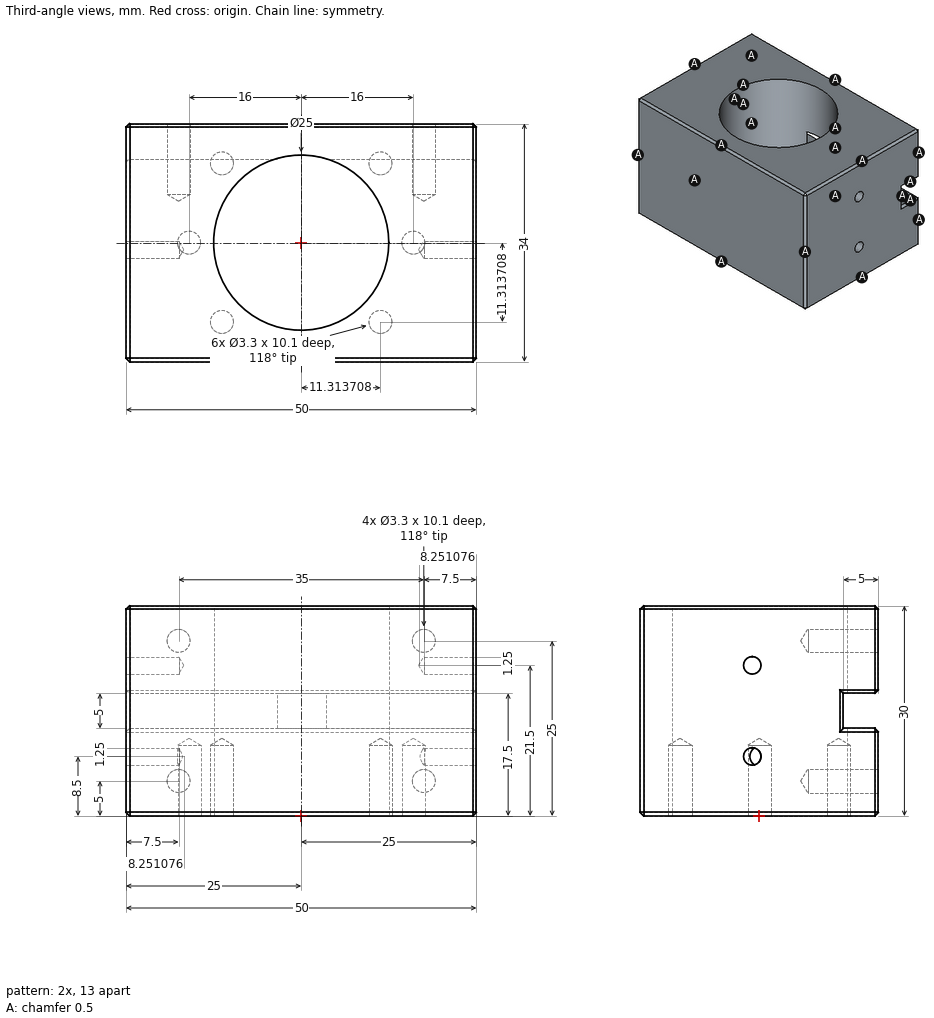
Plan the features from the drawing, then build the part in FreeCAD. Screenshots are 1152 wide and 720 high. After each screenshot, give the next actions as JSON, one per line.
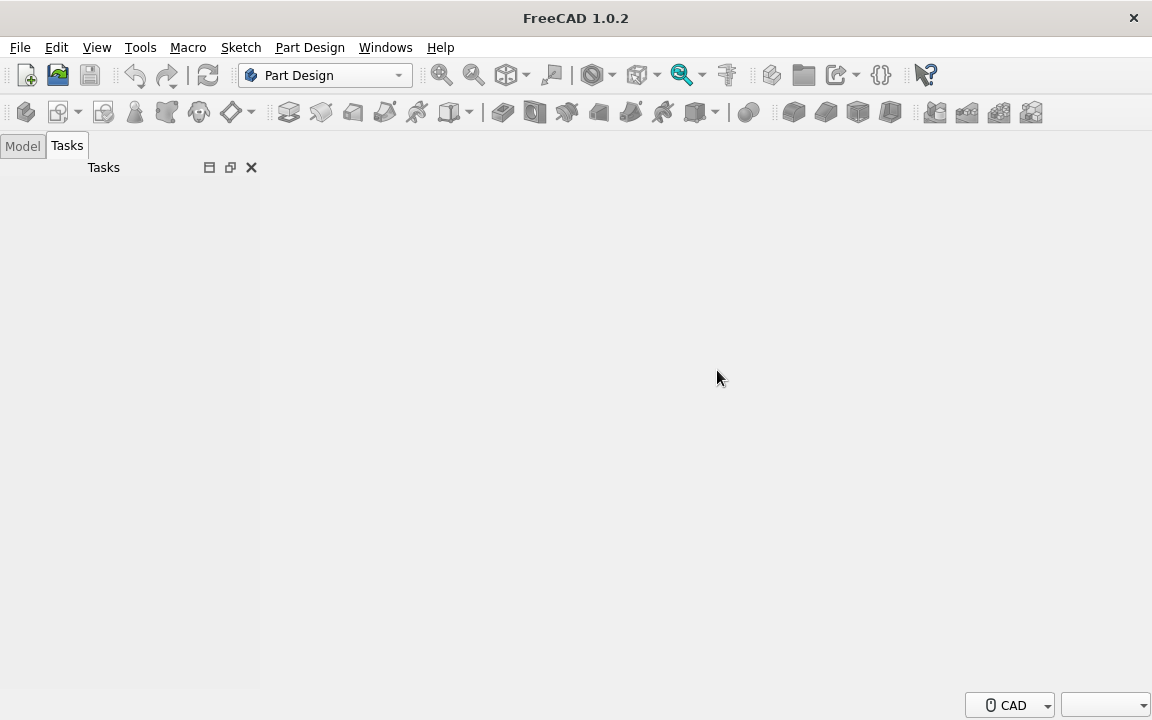
{"action": "key", "text": "ctrl+n"}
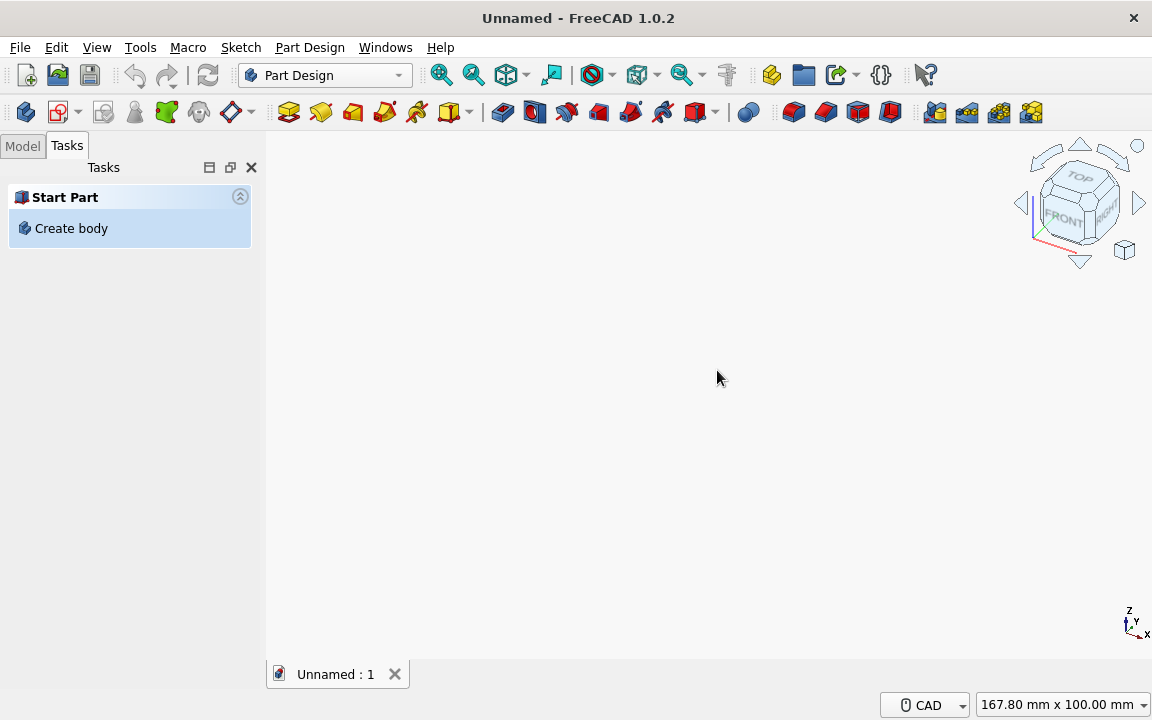
{"action": "left_click", "coordinate": [58, 112]}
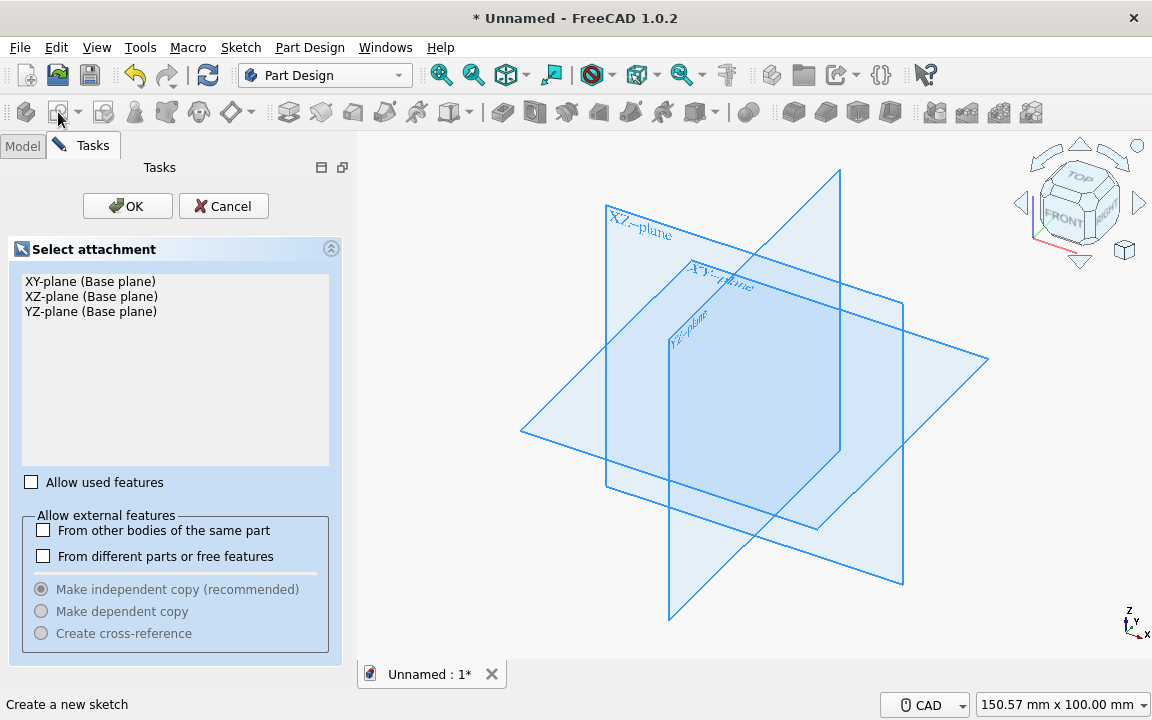
{"action": "left_click", "coordinate": [82, 282]}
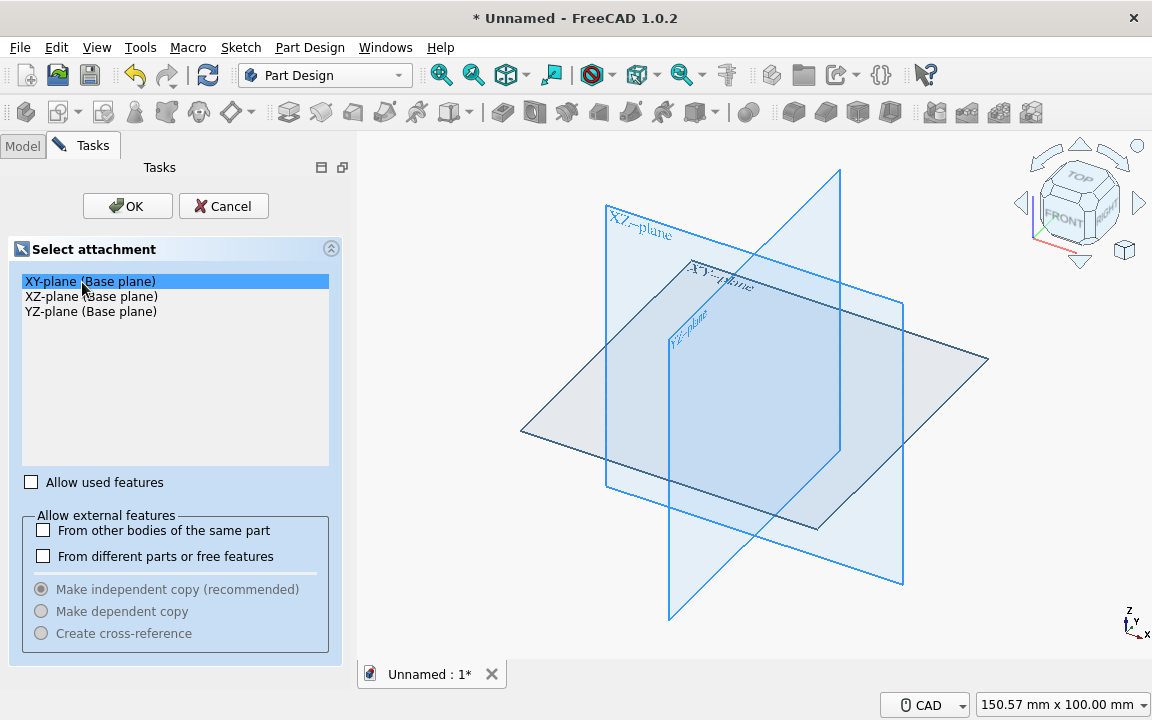
{"action": "left_click", "coordinate": [128, 206]}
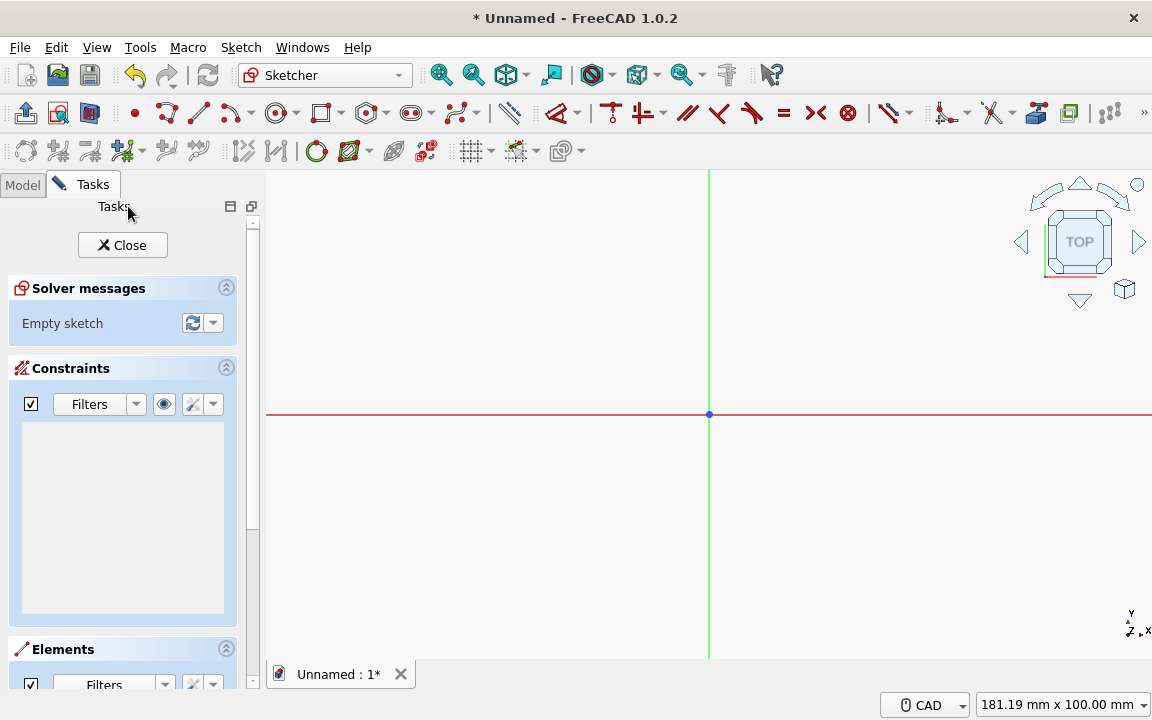
{"action": "scroll", "coordinate": [792, 415], "scroll_direction": "up", "scroll_amount": 3}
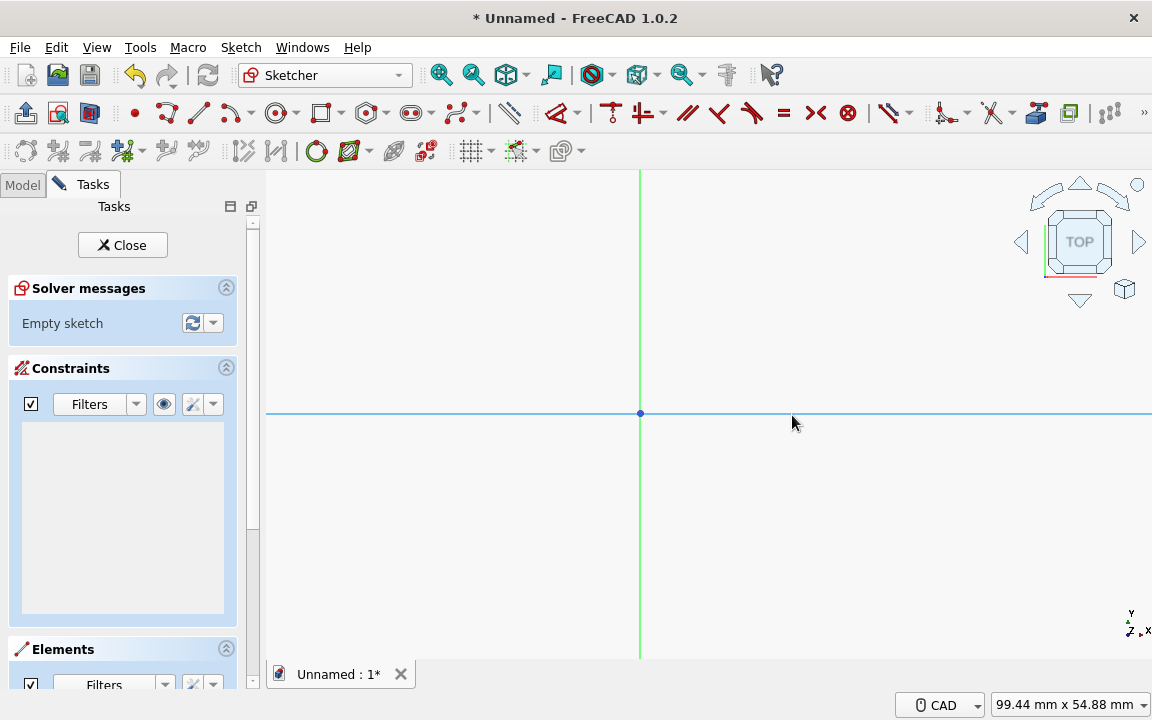
{"action": "left_click", "coordinate": [344, 114]}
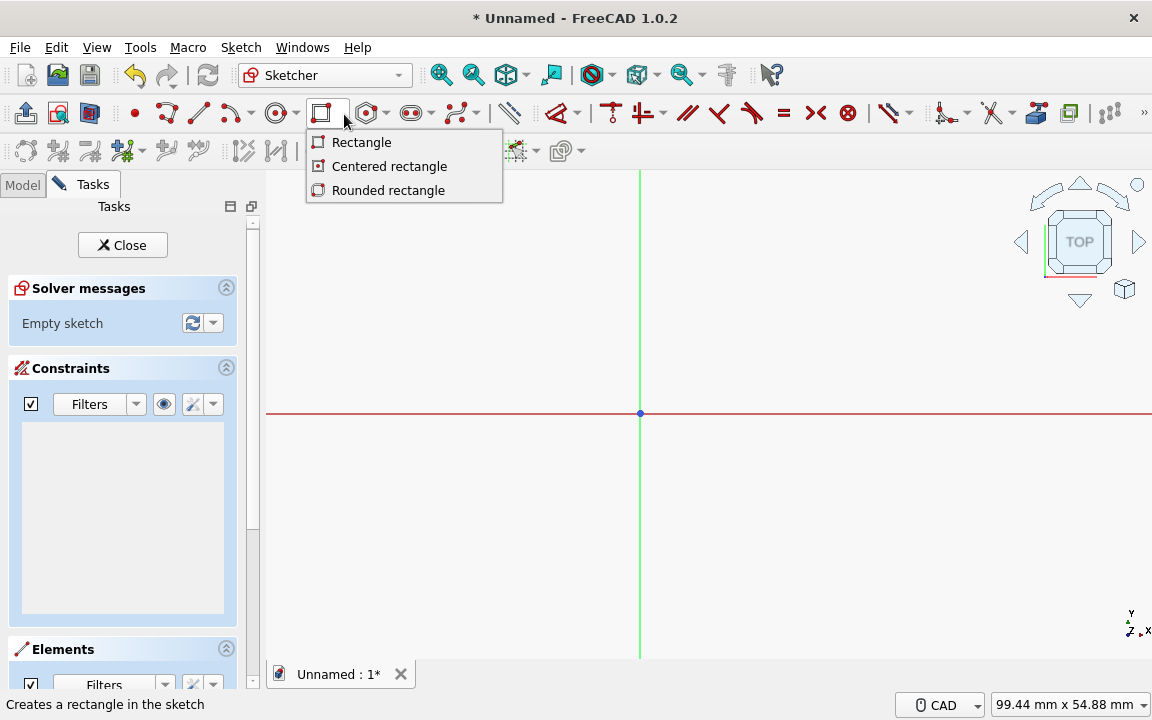
{"action": "left_click", "coordinate": [404, 166]}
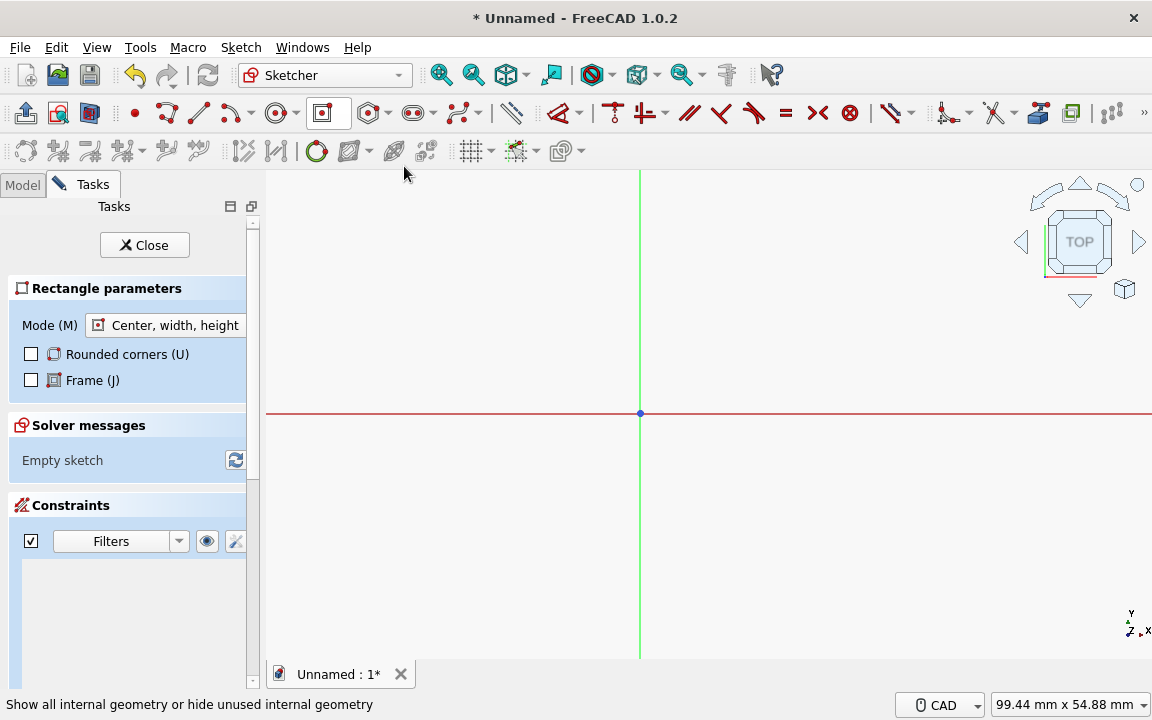
{"action": "left_click", "coordinate": [640, 414]}
{"action": "mouse_move", "coordinate": [863, 262]}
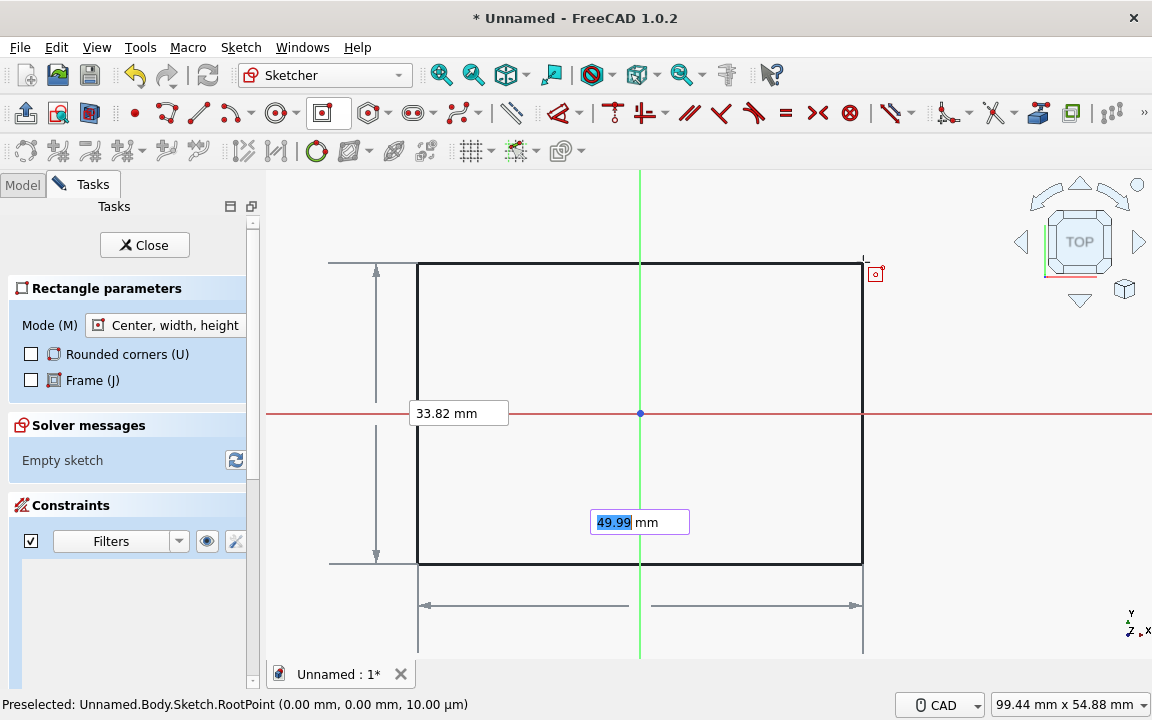
{"action": "type", "text": "50"}
{"action": "key", "text": "Tab"}
{"action": "type", "text": "34"}
{"action": "key", "text": "Return"}
{"action": "key", "text": "Escape"}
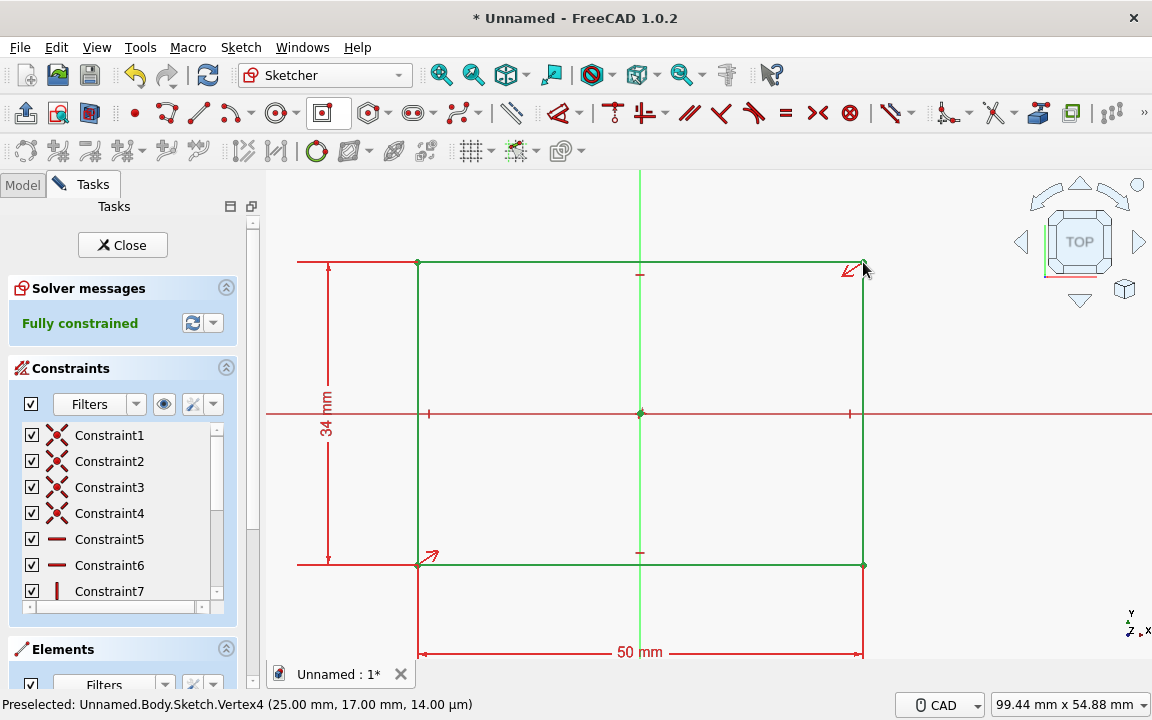
{"action": "left_click", "coordinate": [123, 245]}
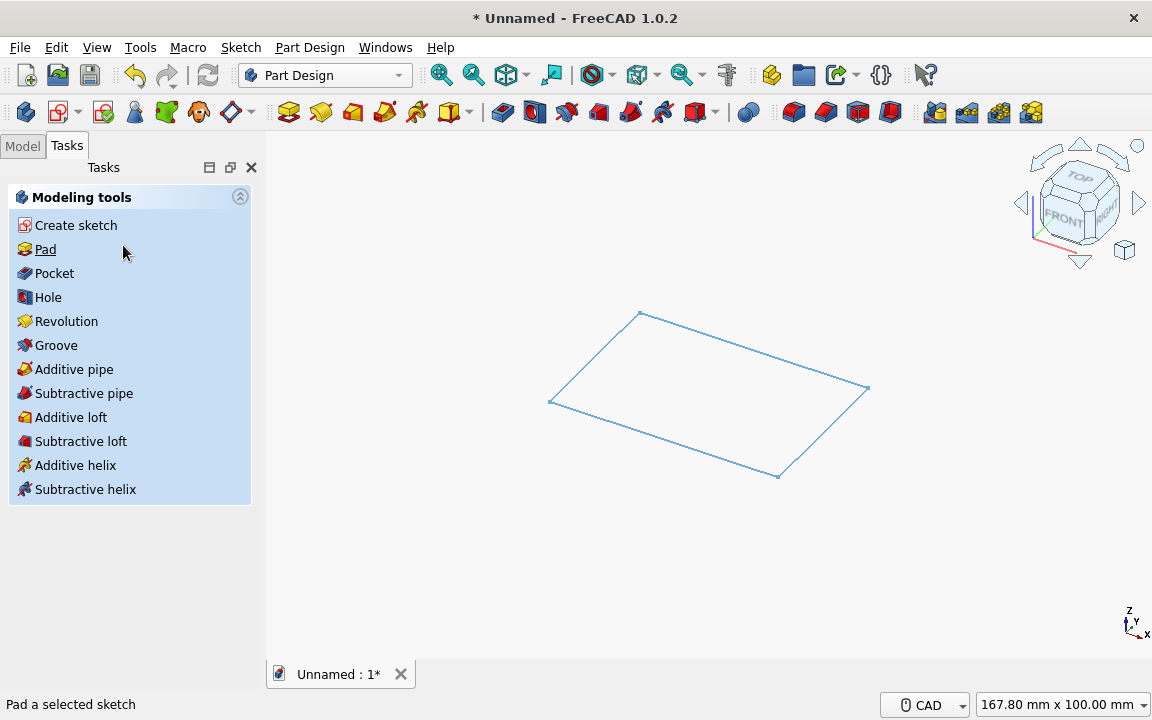
{"action": "left_click", "coordinate": [290, 112]}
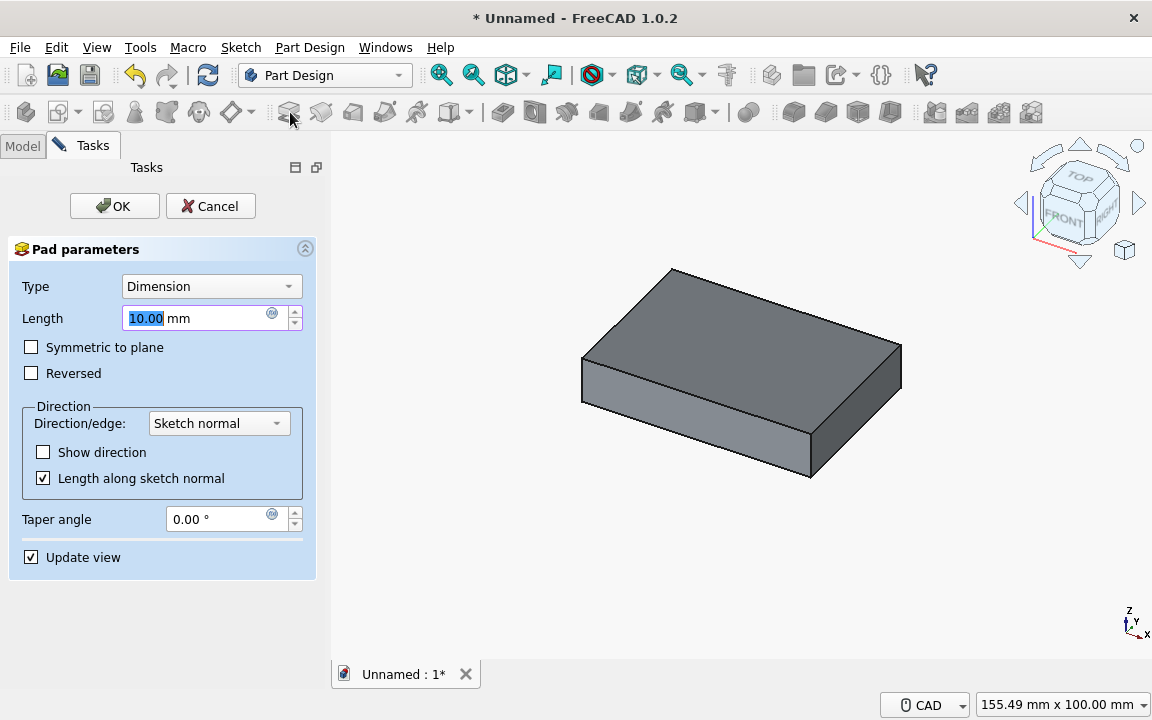
{"action": "type", "text": "30"}
{"action": "key", "text": "Tab"}